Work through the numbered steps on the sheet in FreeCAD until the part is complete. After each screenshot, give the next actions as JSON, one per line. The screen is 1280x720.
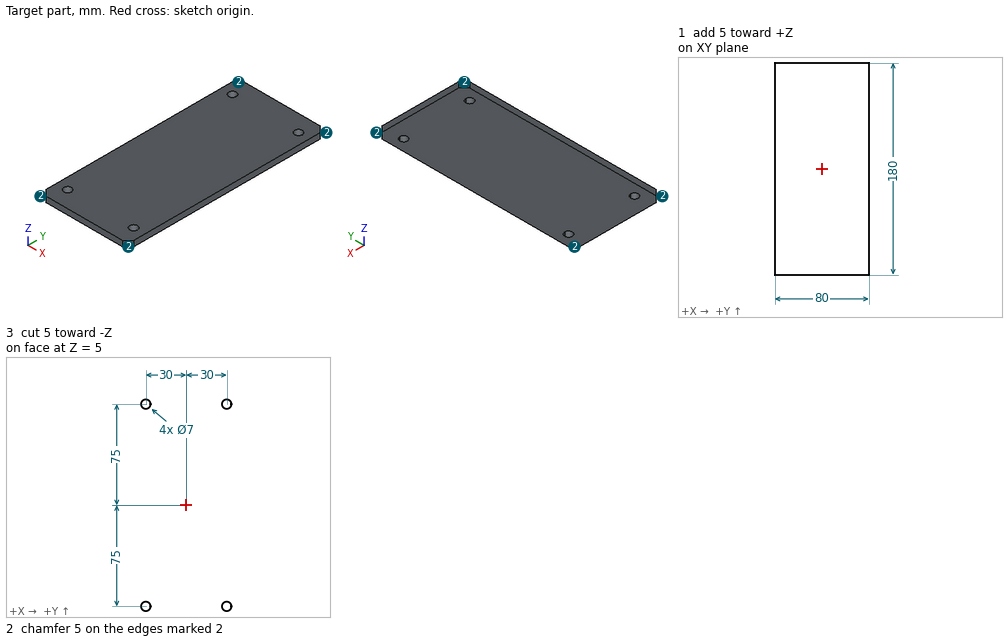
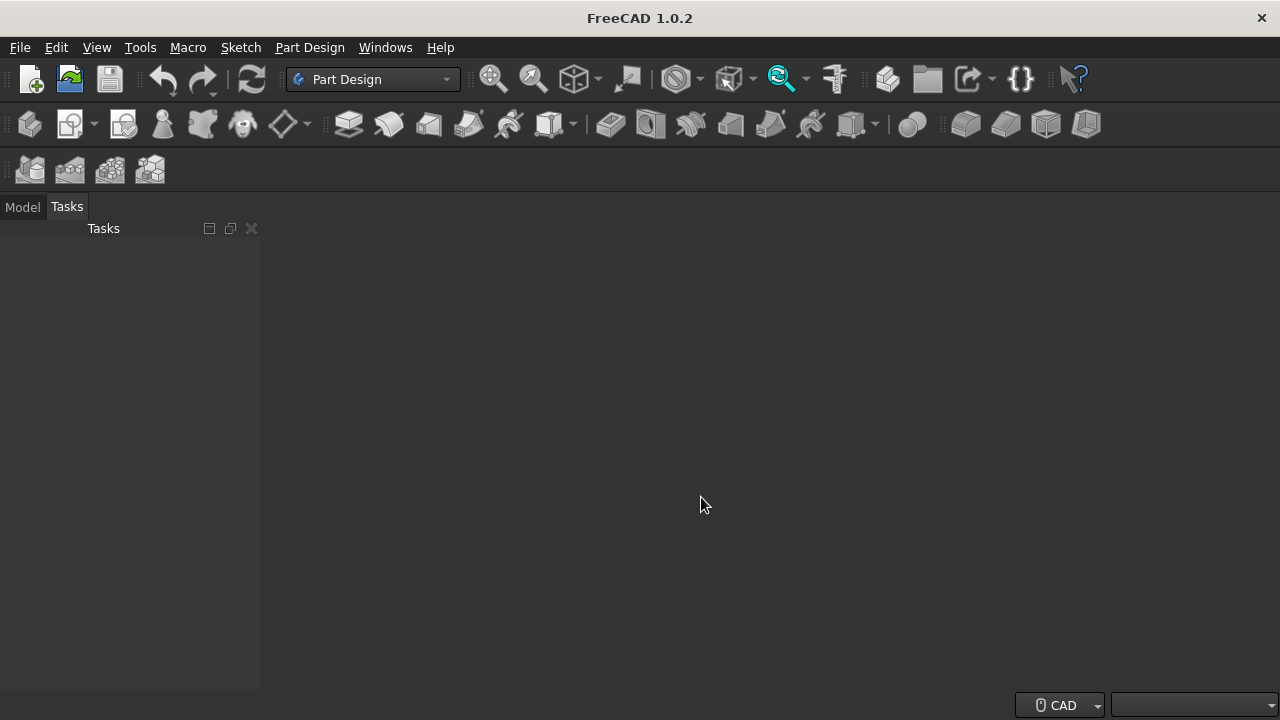
{"action": "left_click", "coordinate": [30, 80]}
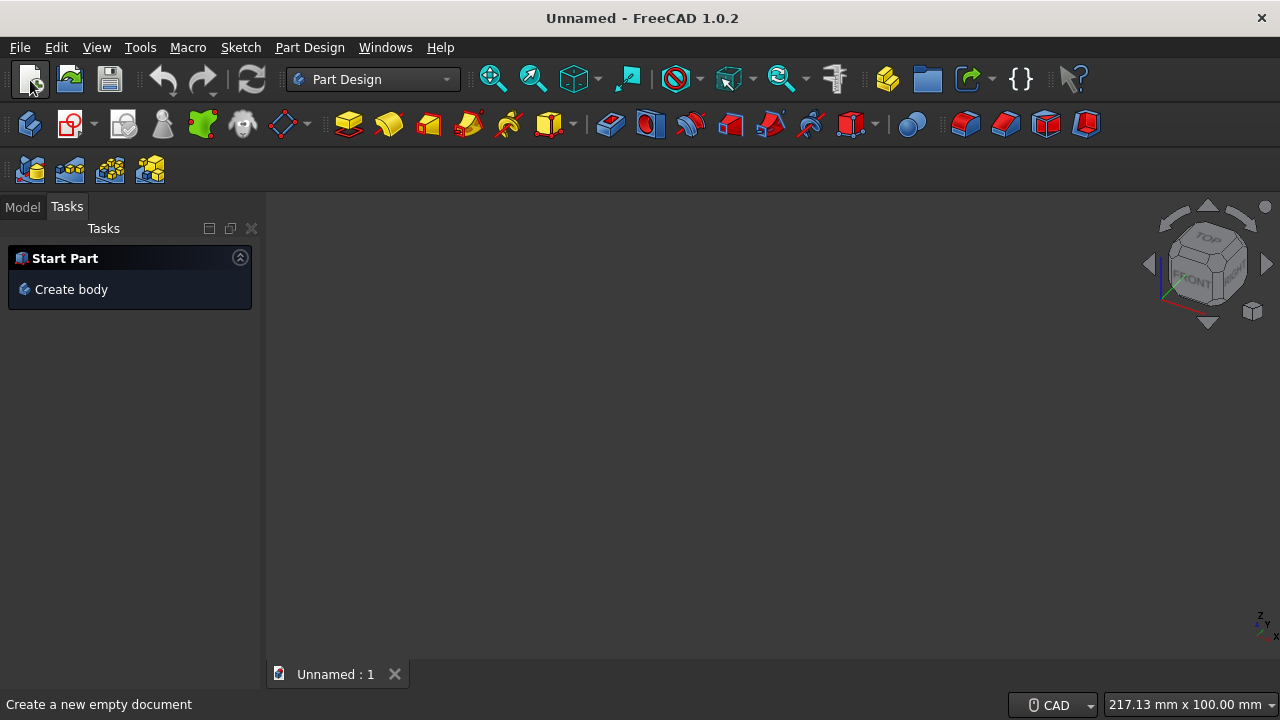
{"action": "left_click", "coordinate": [70, 124]}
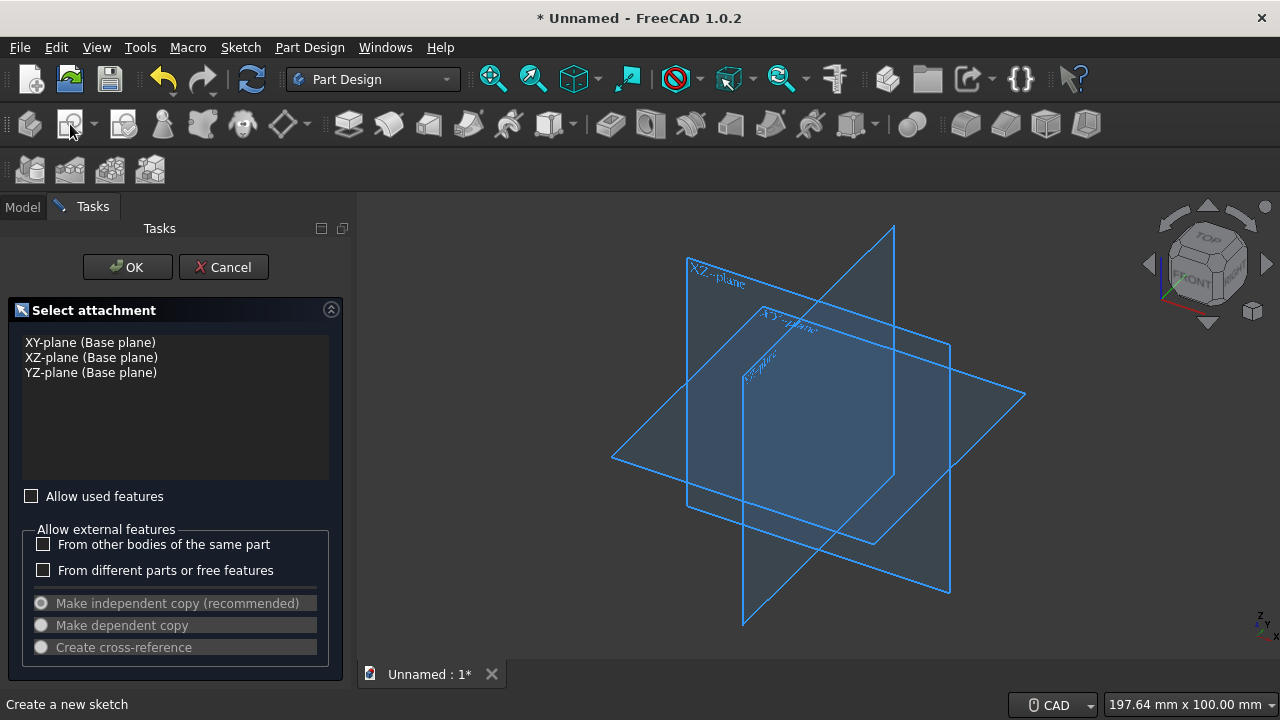
{"action": "left_click", "coordinate": [82, 342]}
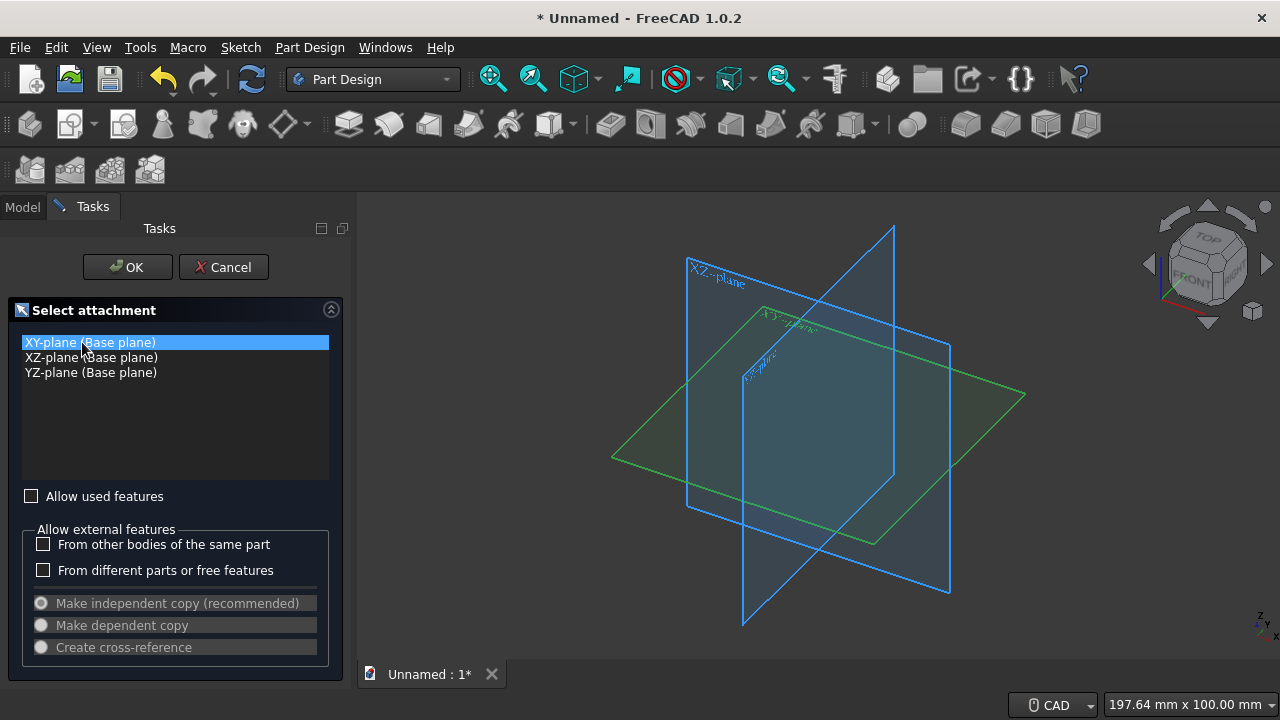
{"action": "left_click", "coordinate": [128, 267]}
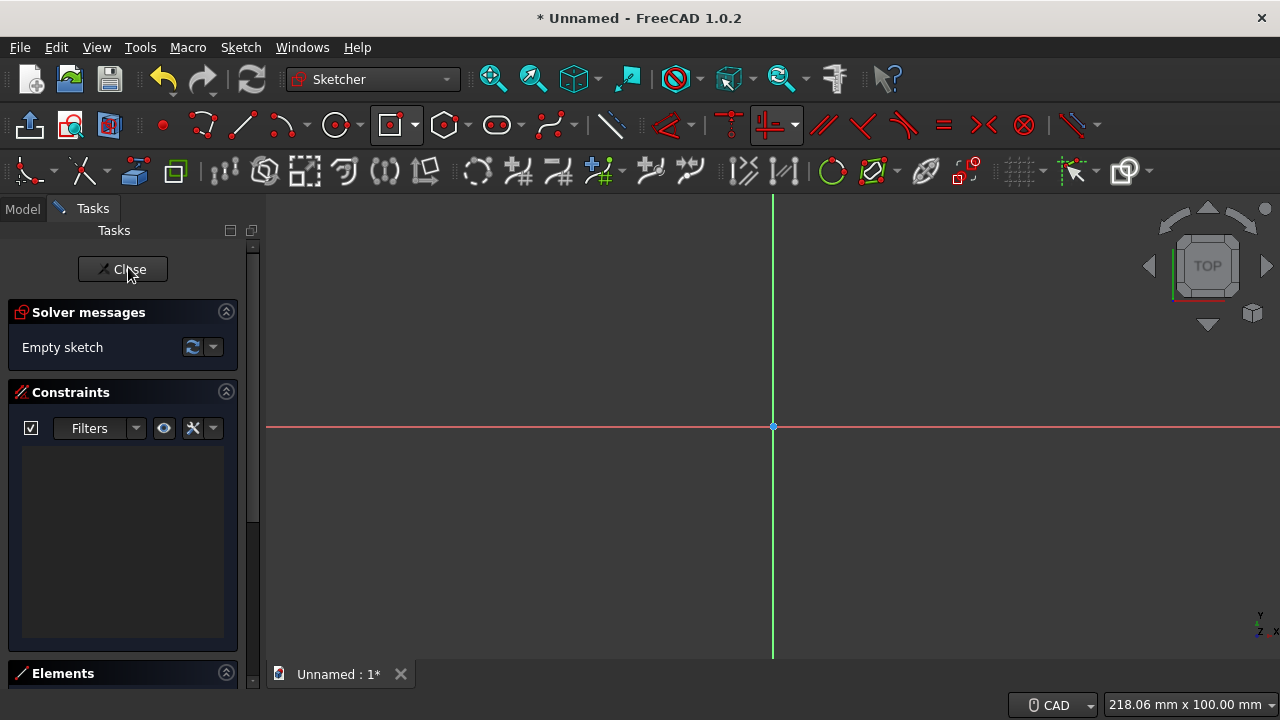
{"action": "scroll", "coordinate": [665, 427], "scroll_direction": "down", "scroll_amount": 5}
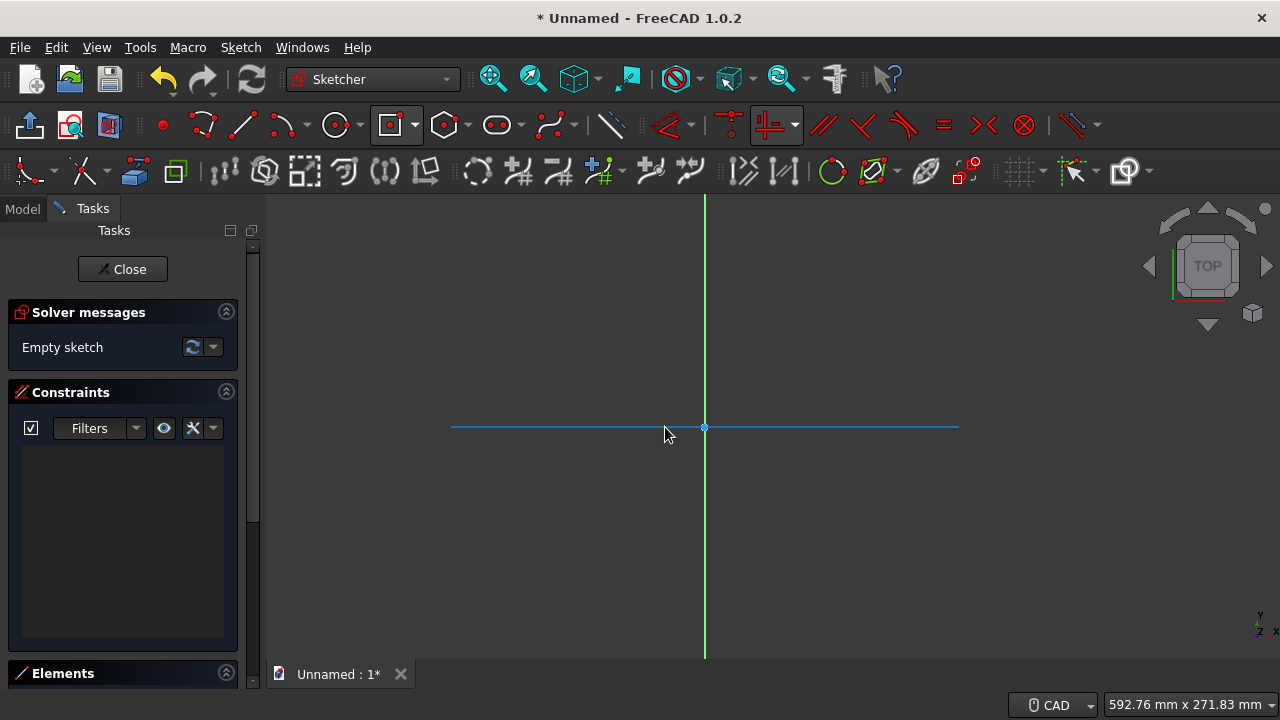
{"action": "left_click", "coordinate": [390, 126]}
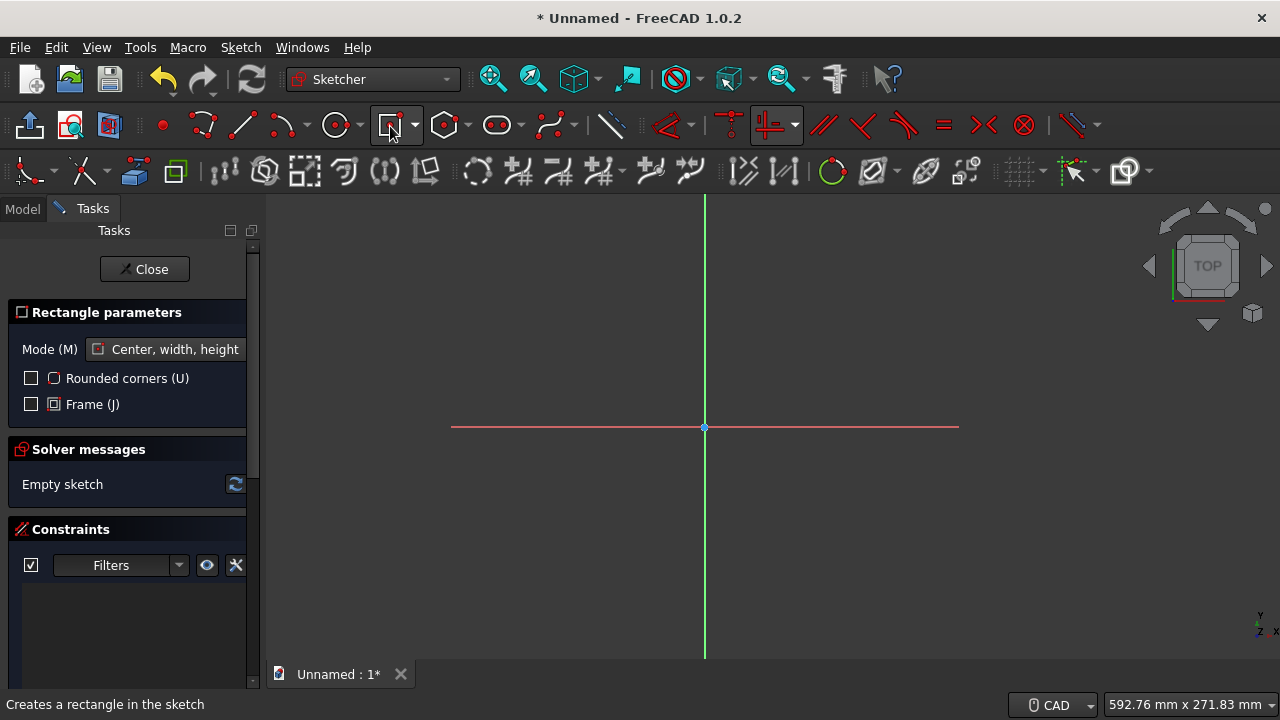
{"action": "left_click", "coordinate": [705, 427]}
{"action": "mouse_move", "coordinate": [773, 273]}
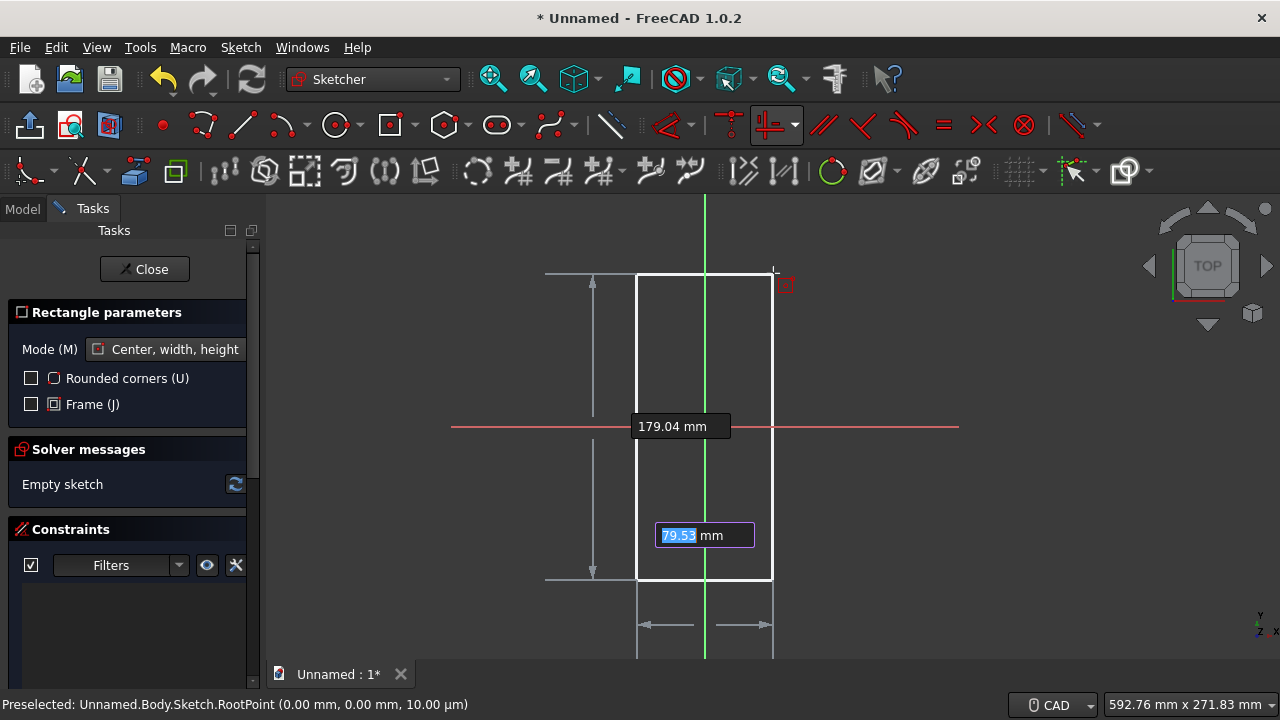
{"action": "type", "text": "80"}
{"action": "key", "text": "Tab"}
{"action": "type", "text": "180"}
{"action": "key", "text": "Return"}
{"action": "key", "text": "Escape"}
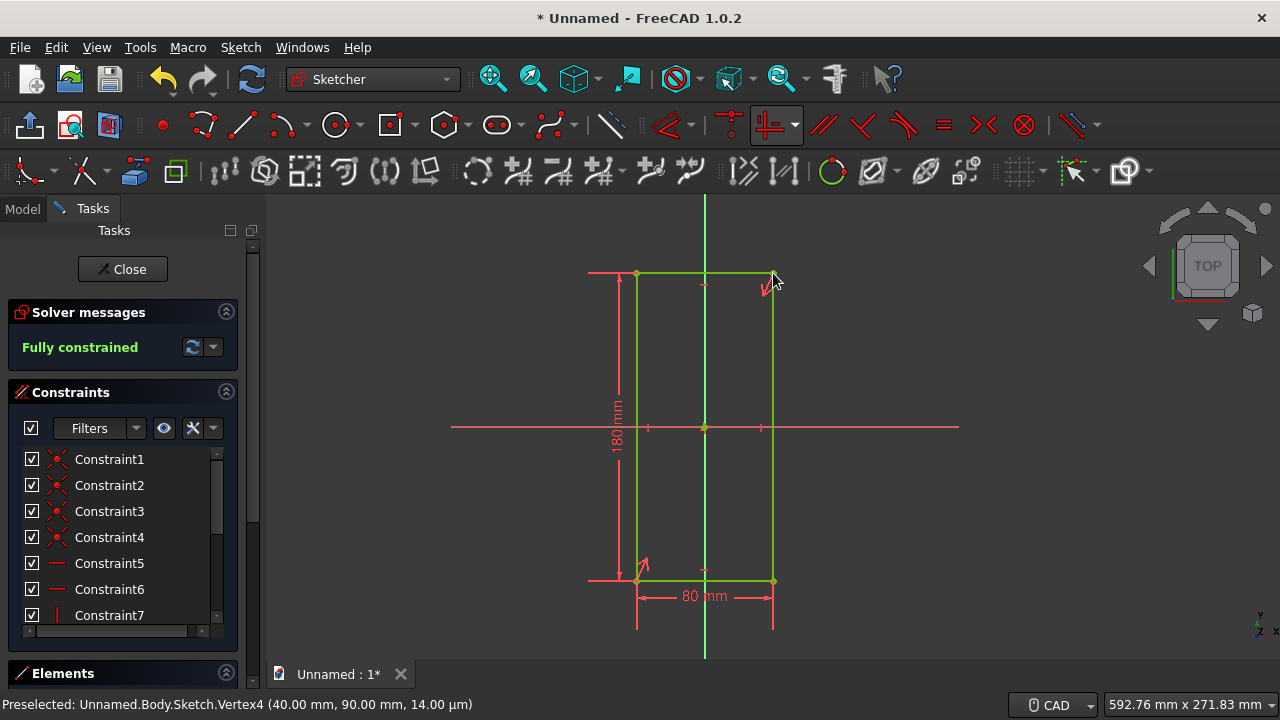
{"action": "left_click", "coordinate": [123, 269]}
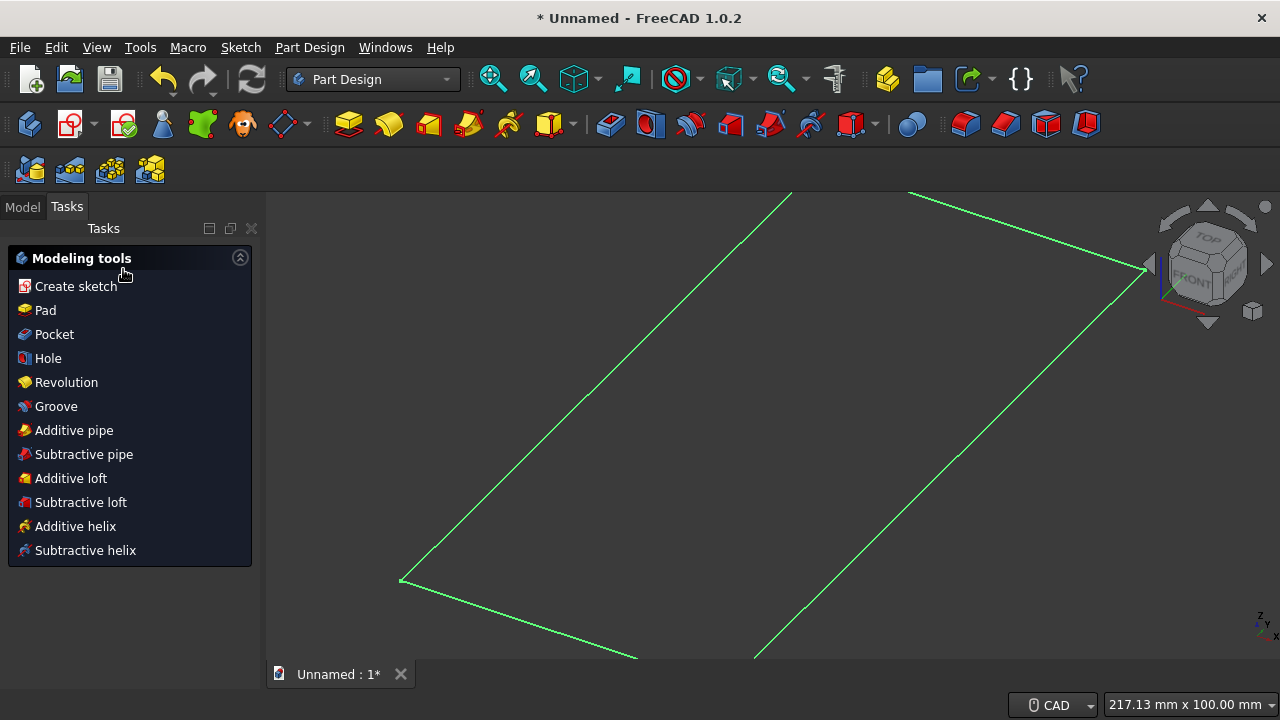
{"action": "left_click", "coordinate": [350, 124]}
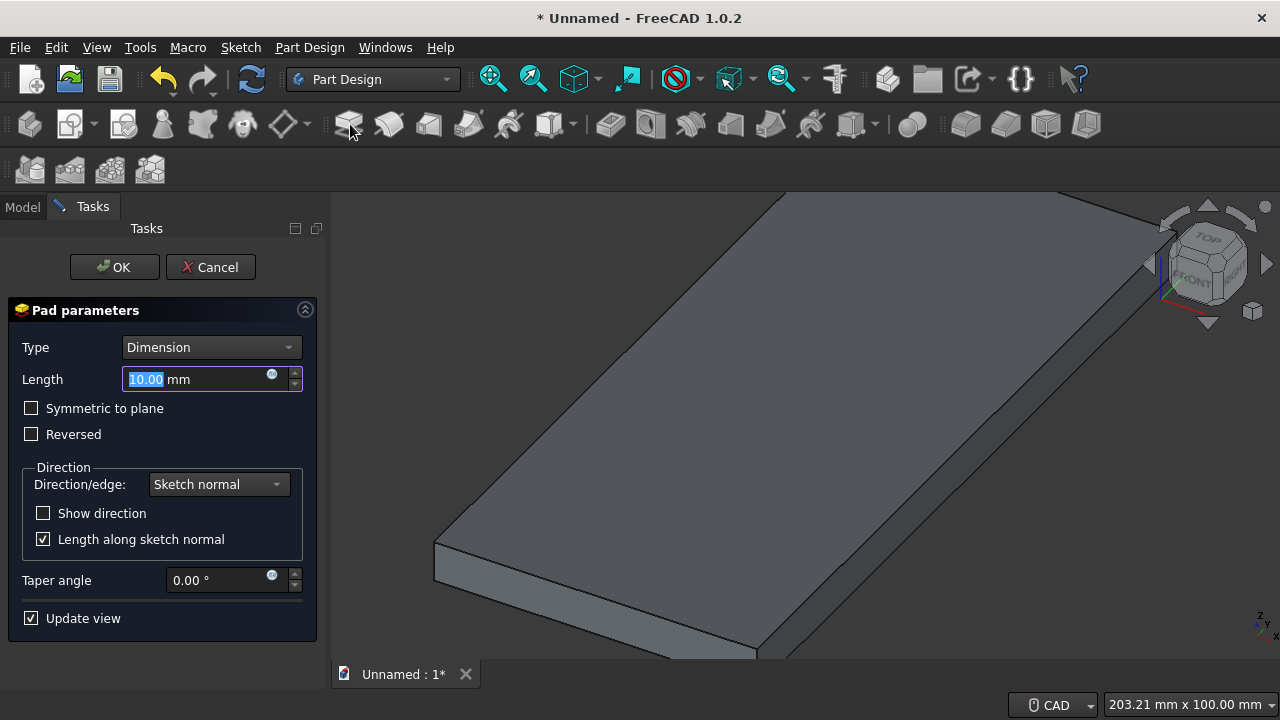
{"action": "type", "text": "5"}
{"action": "key", "text": "Tab"}